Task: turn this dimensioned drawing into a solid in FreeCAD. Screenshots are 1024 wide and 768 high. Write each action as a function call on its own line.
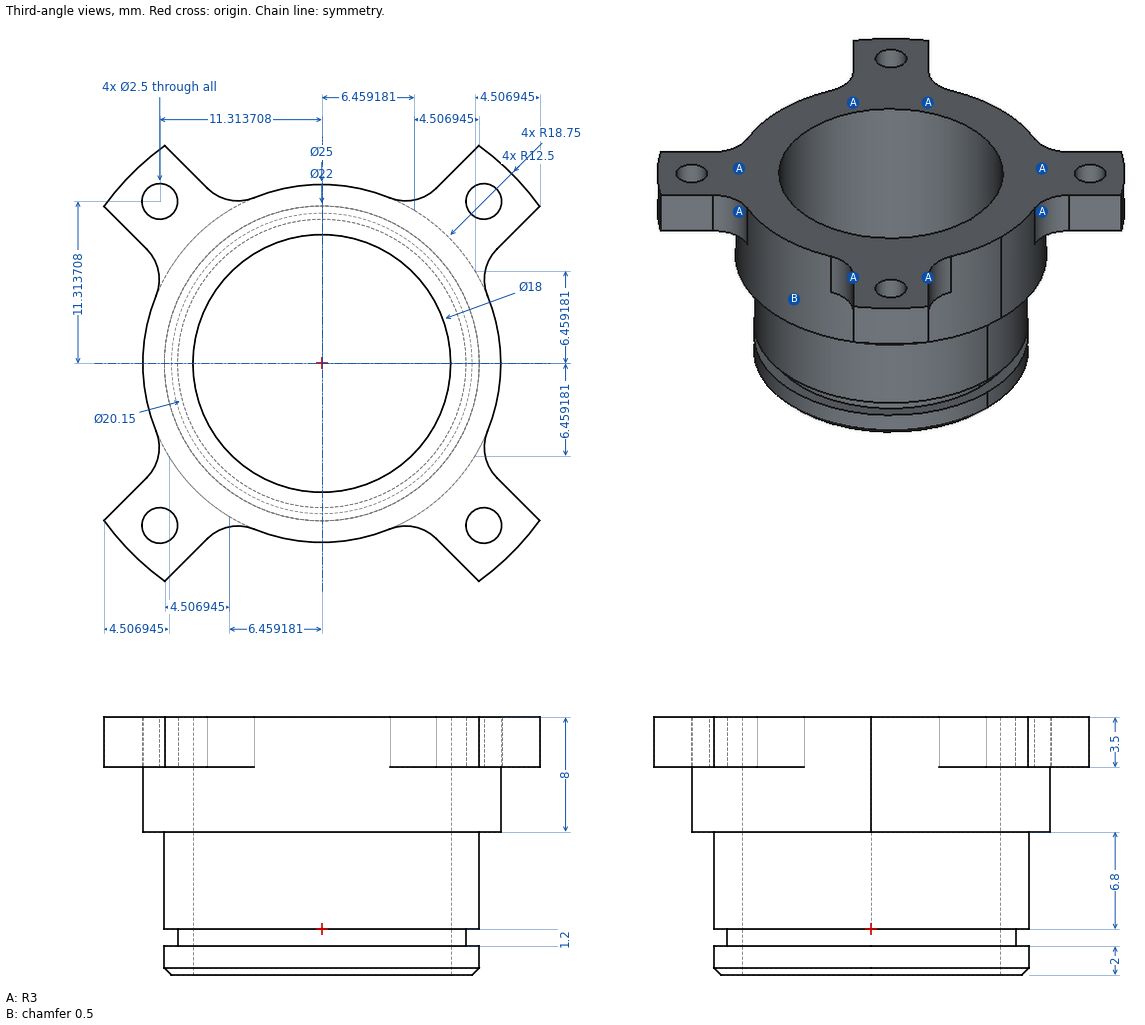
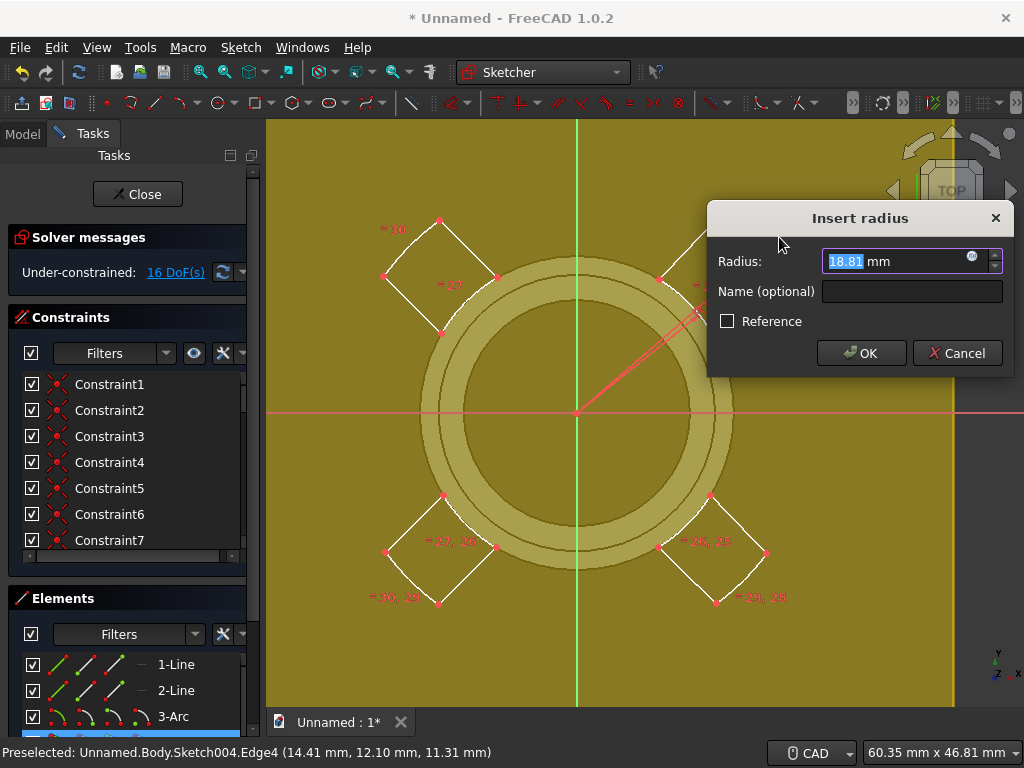
text(18.75)
key(Return)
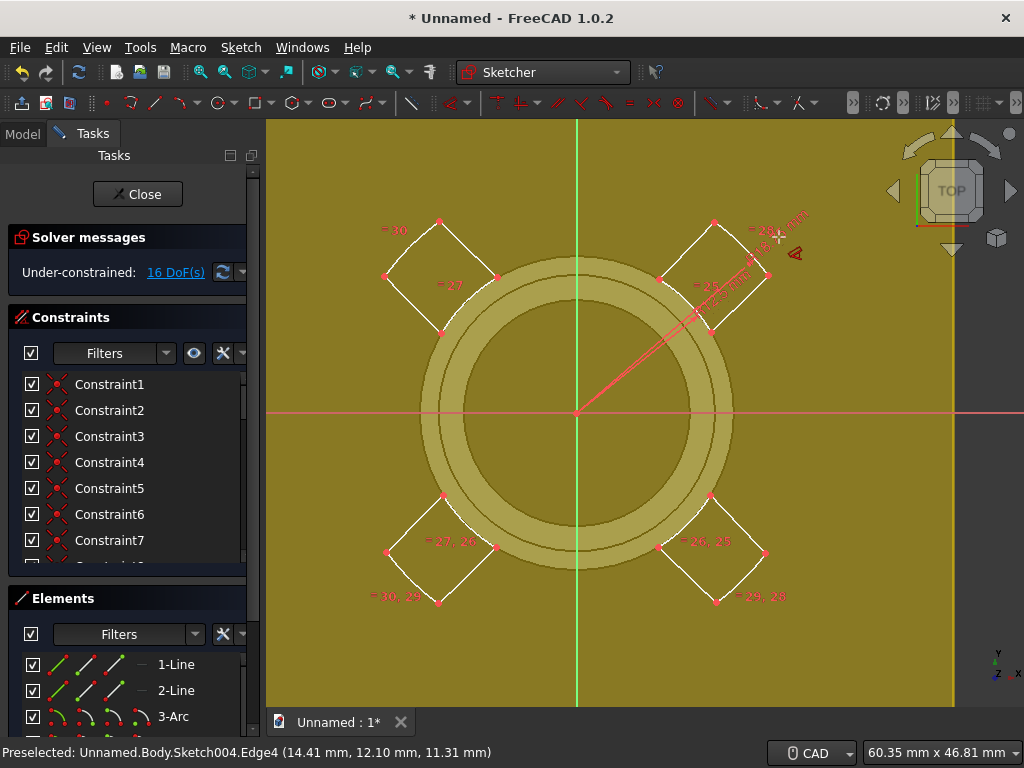
click(659, 279)
click(618, 245)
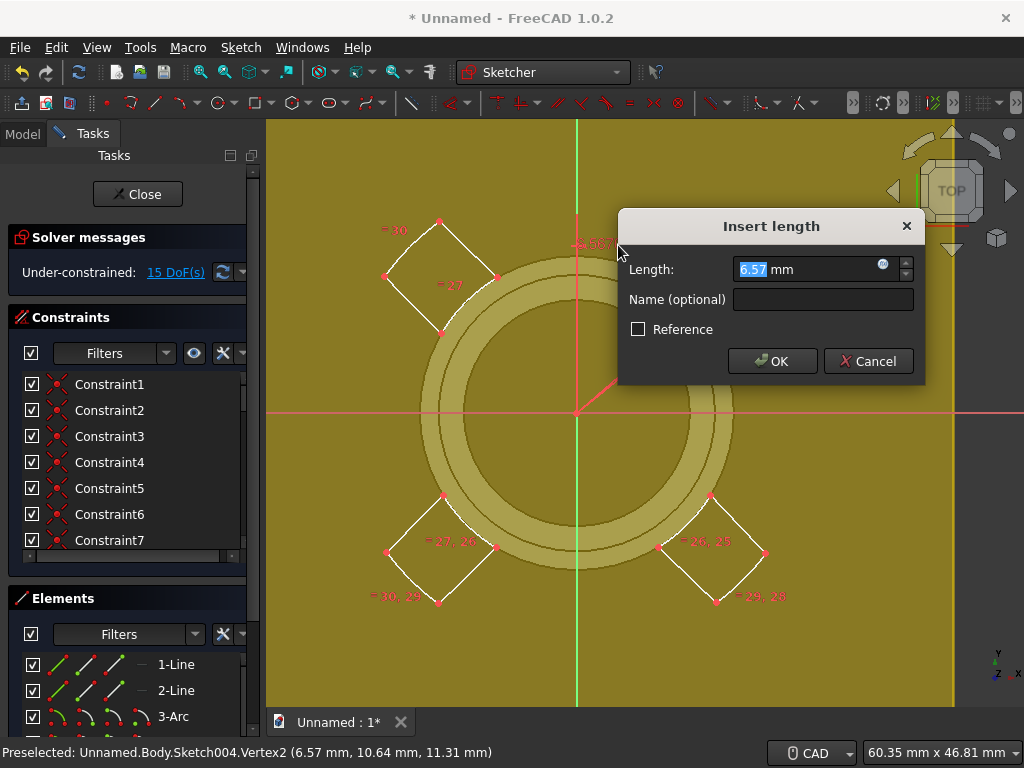
text(6.459181)
key(Return)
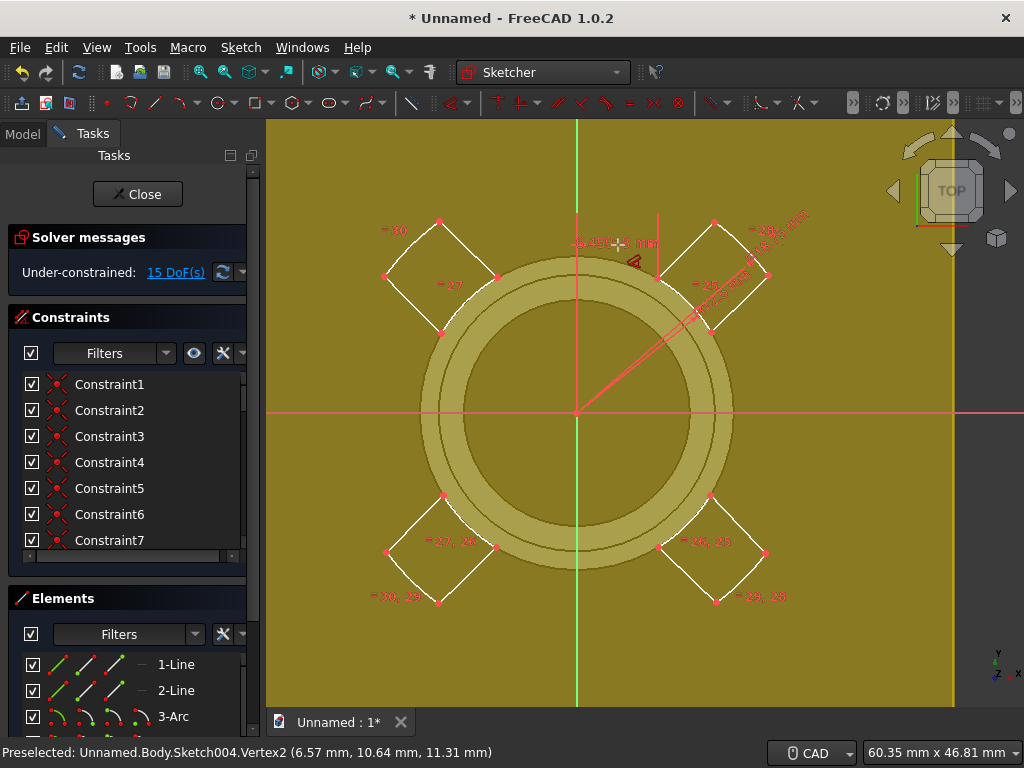
click(712, 332)
click(746, 373)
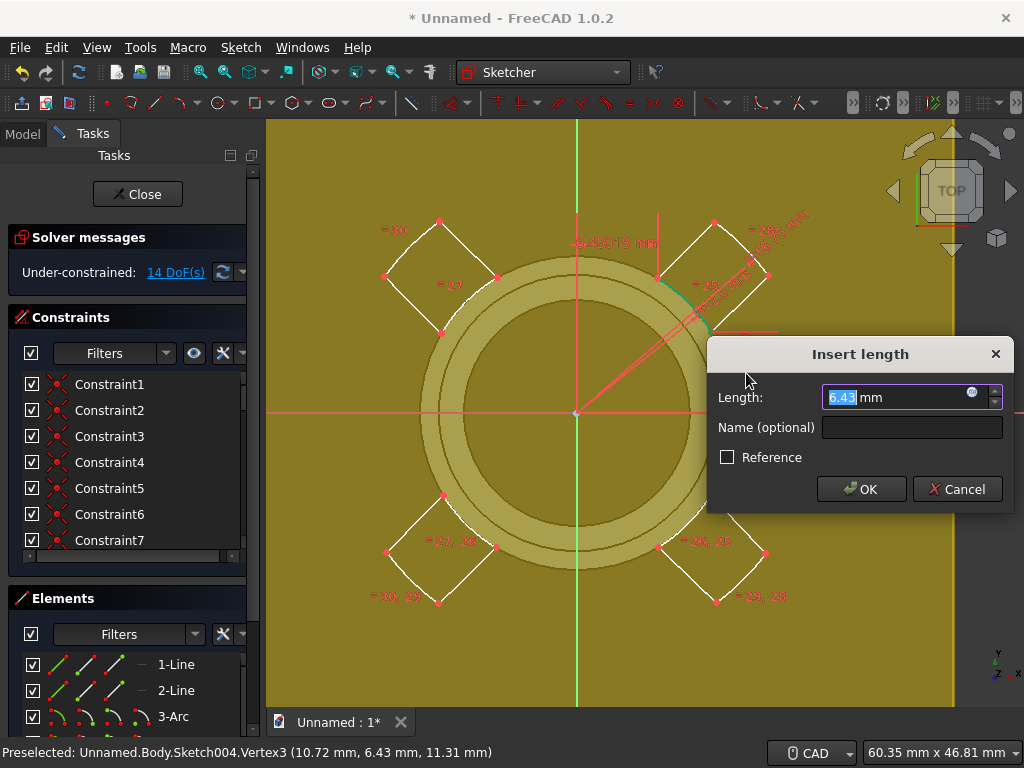
text(6.459181)
key(Return)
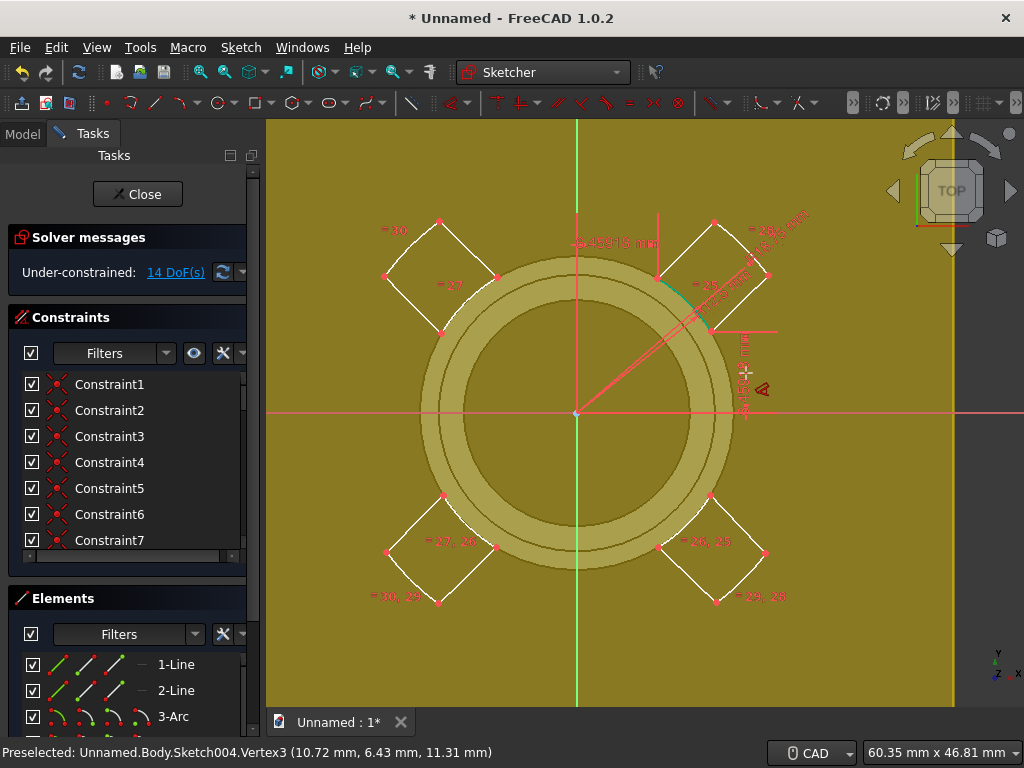
click(711, 495)
click(745, 454)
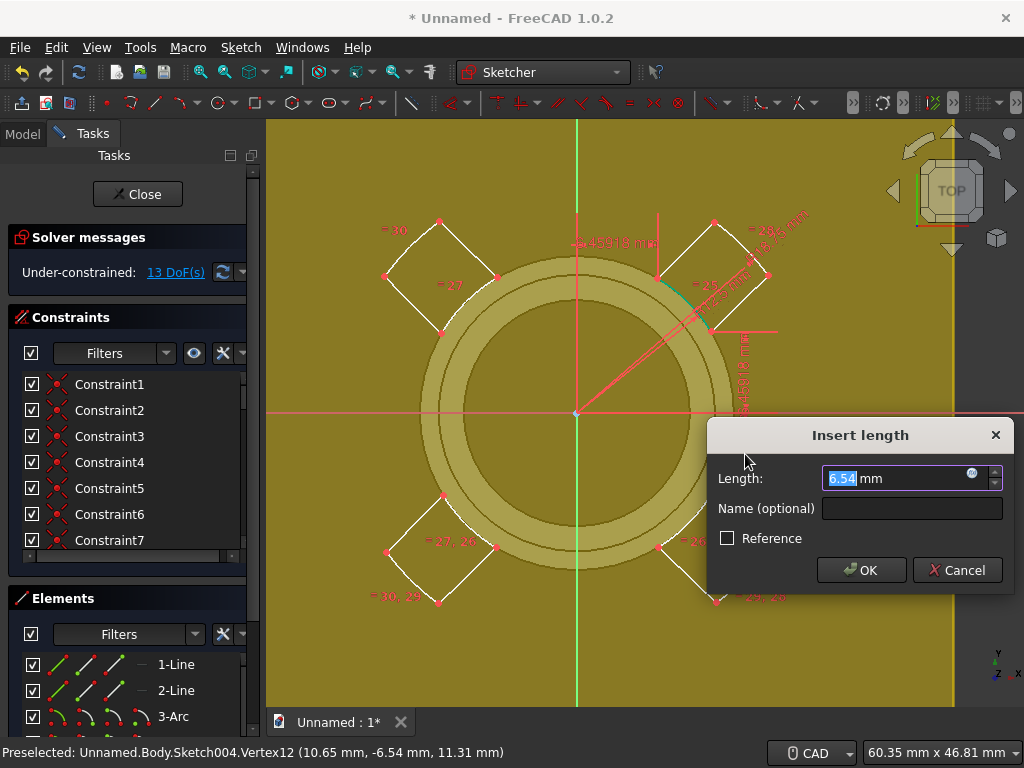
text(6.459181)
key(Return)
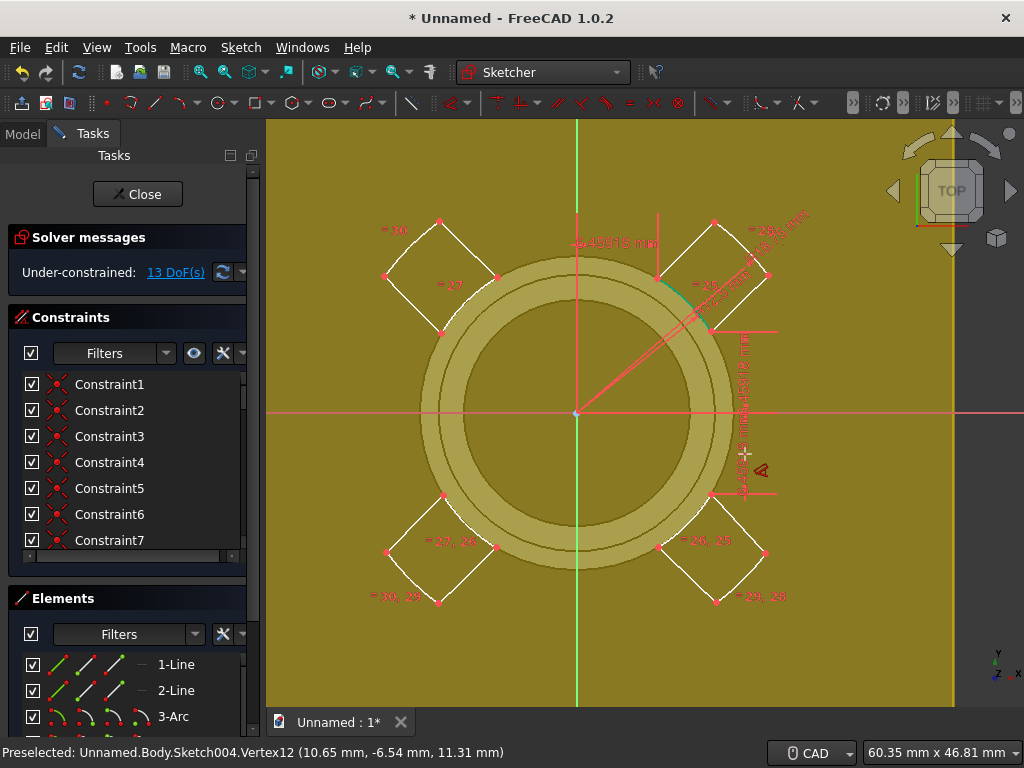
click(658, 547)
click(618, 581)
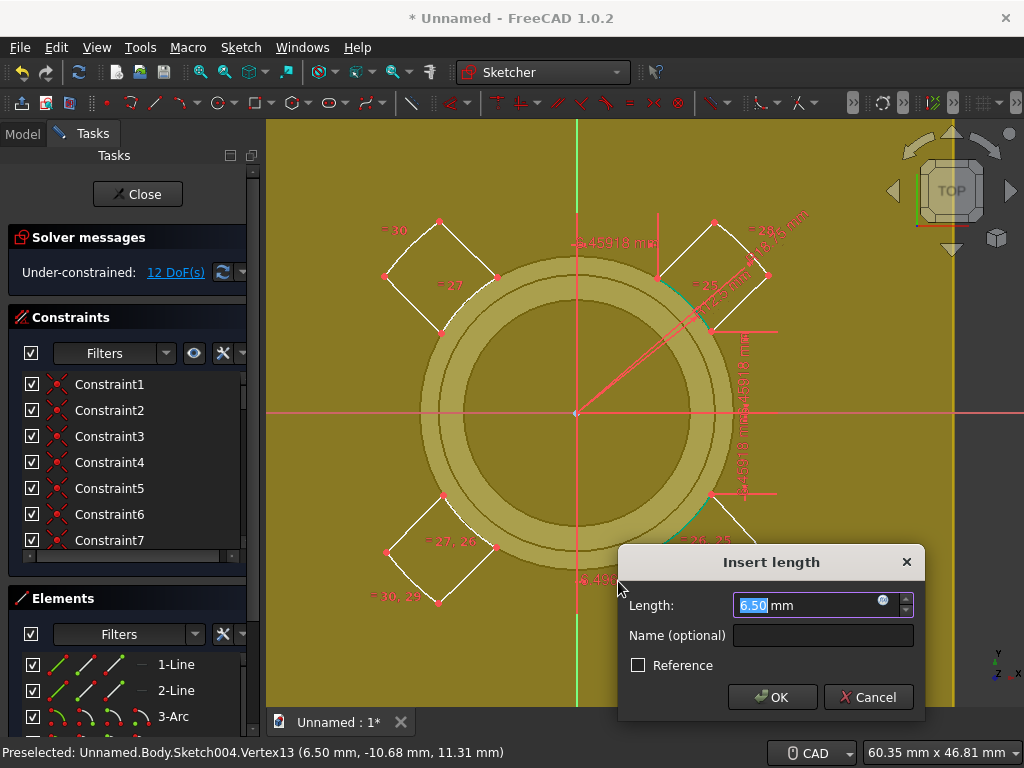
text(6.459181)
key(Return)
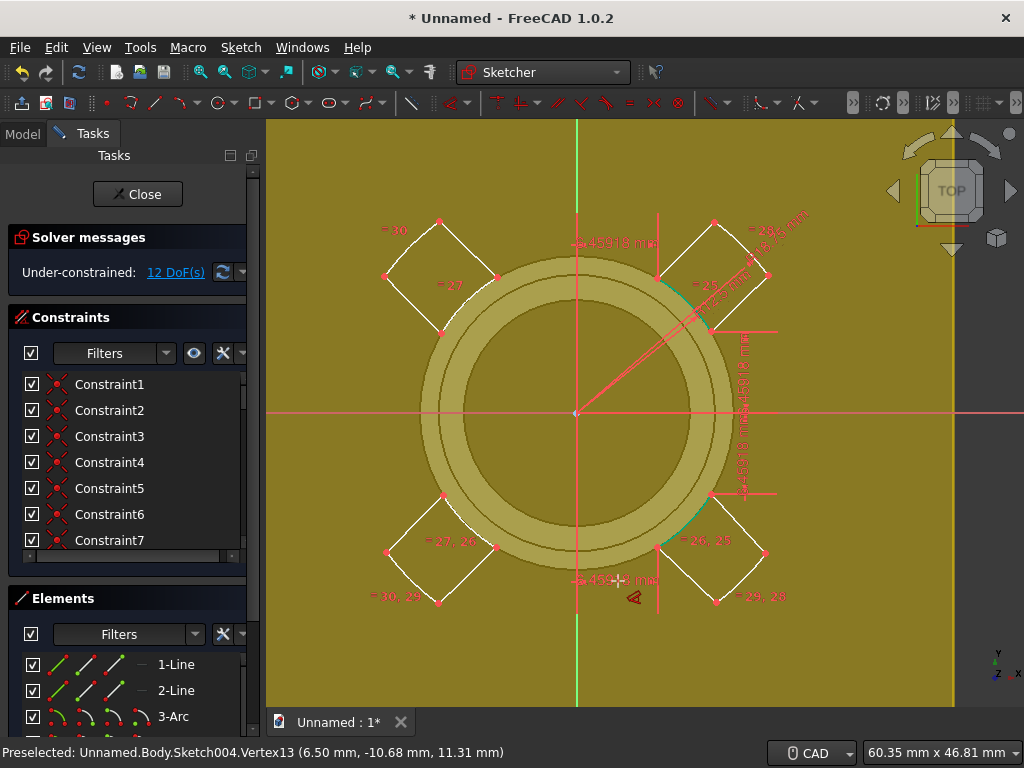
click(496, 548)
click(536, 582)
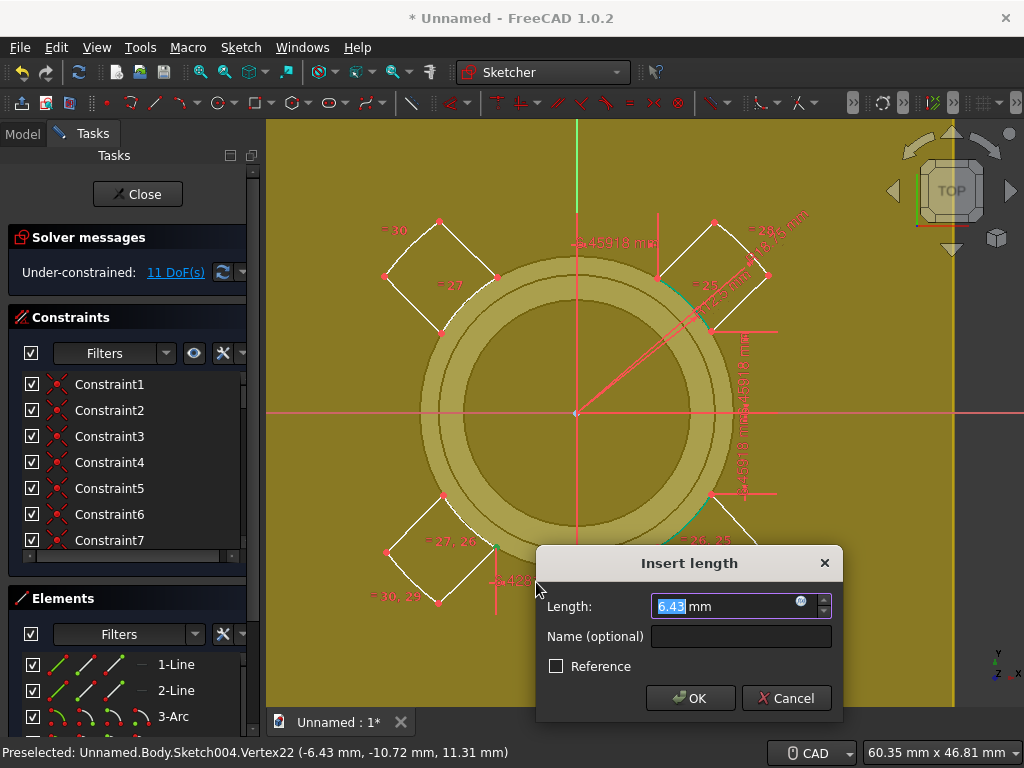
text(6.459181)
key(Return)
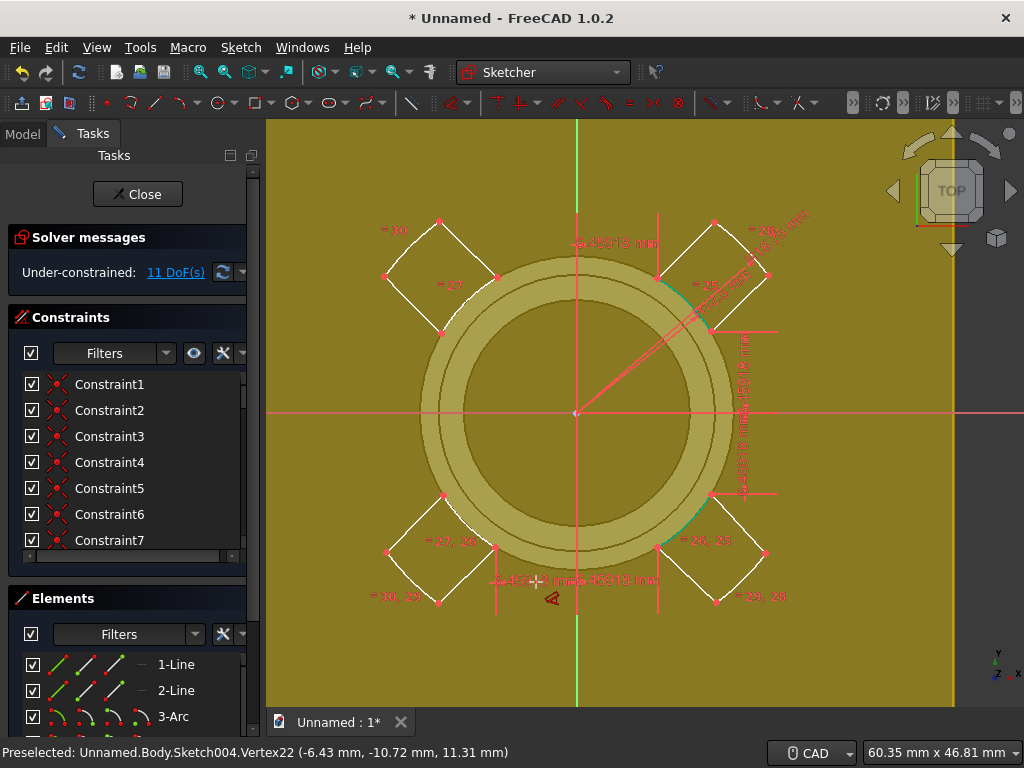
click(443, 495)
click(409, 454)